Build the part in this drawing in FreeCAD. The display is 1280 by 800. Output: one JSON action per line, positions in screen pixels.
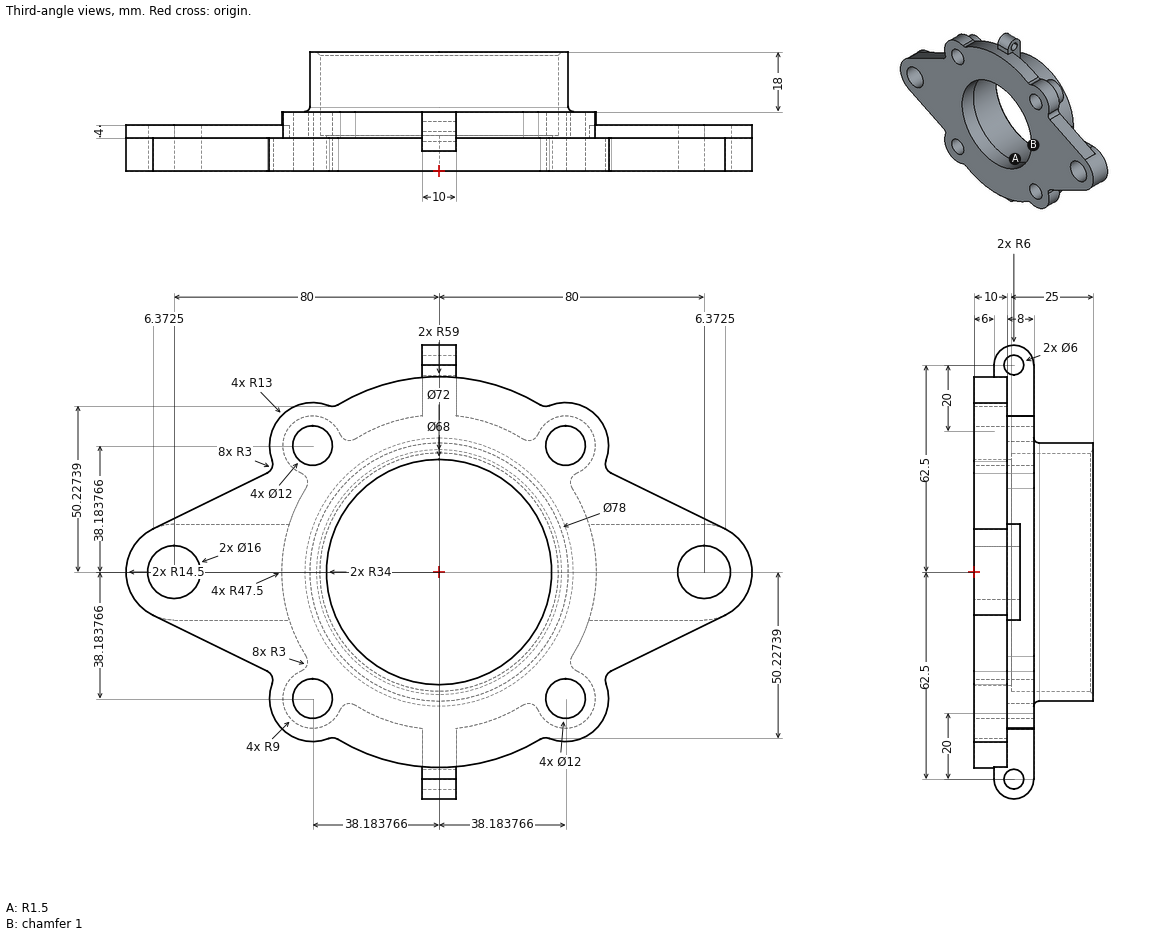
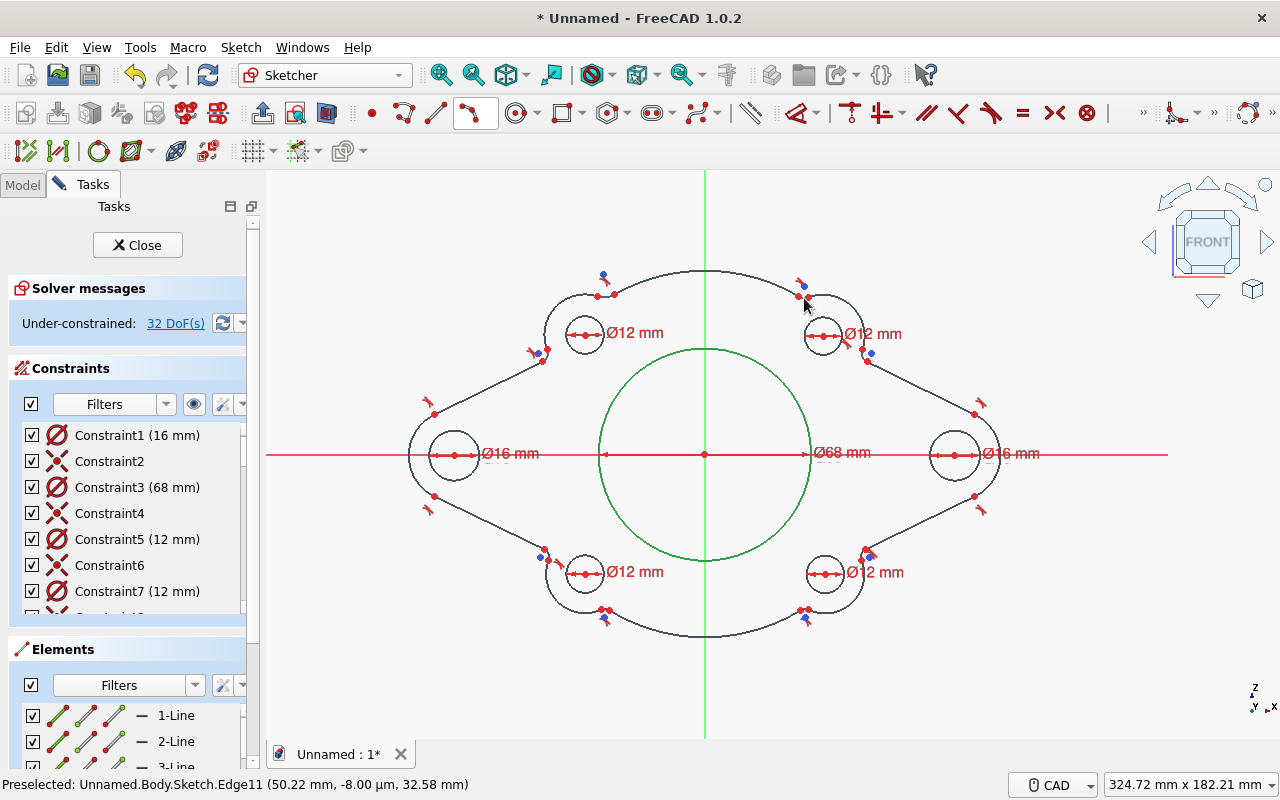
{"action": "scroll", "coordinate": [863, 552], "scroll_direction": "up", "scroll_amount": 7}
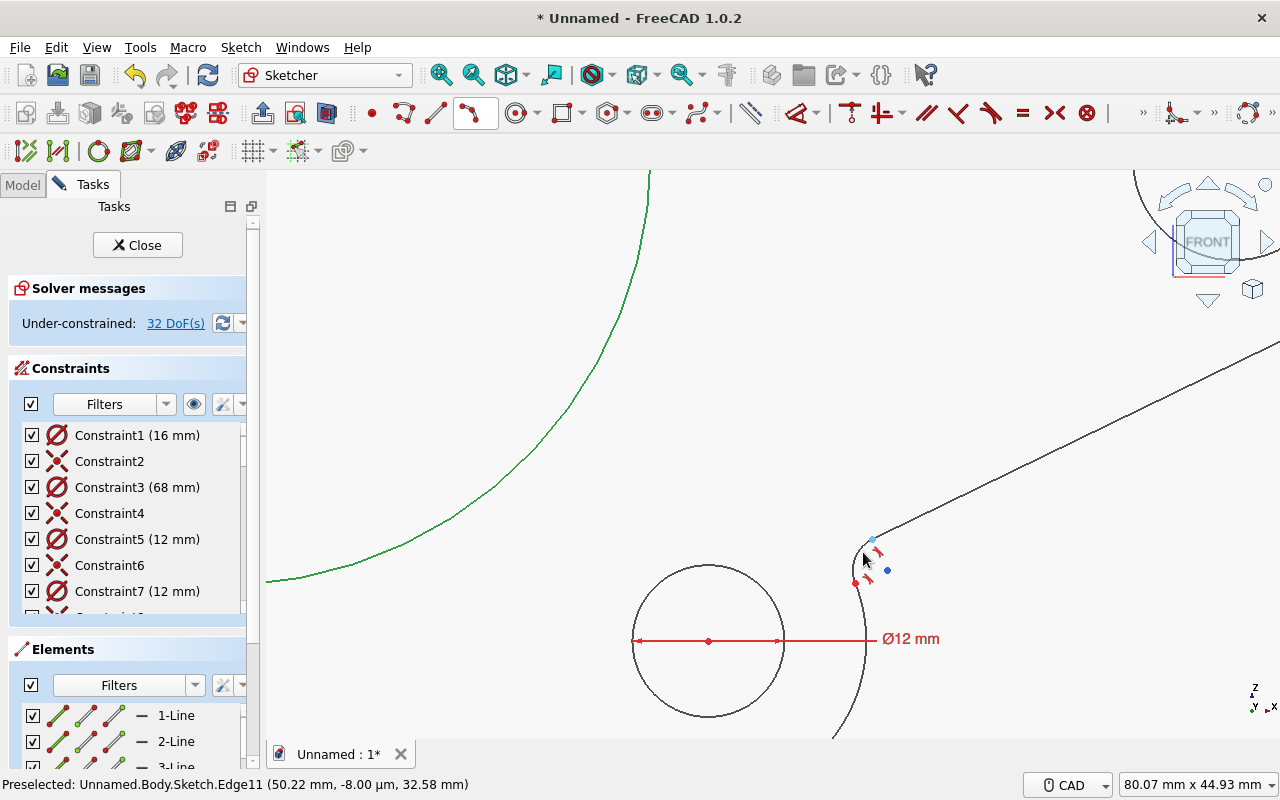
{"action": "left_click", "coordinate": [860, 549]}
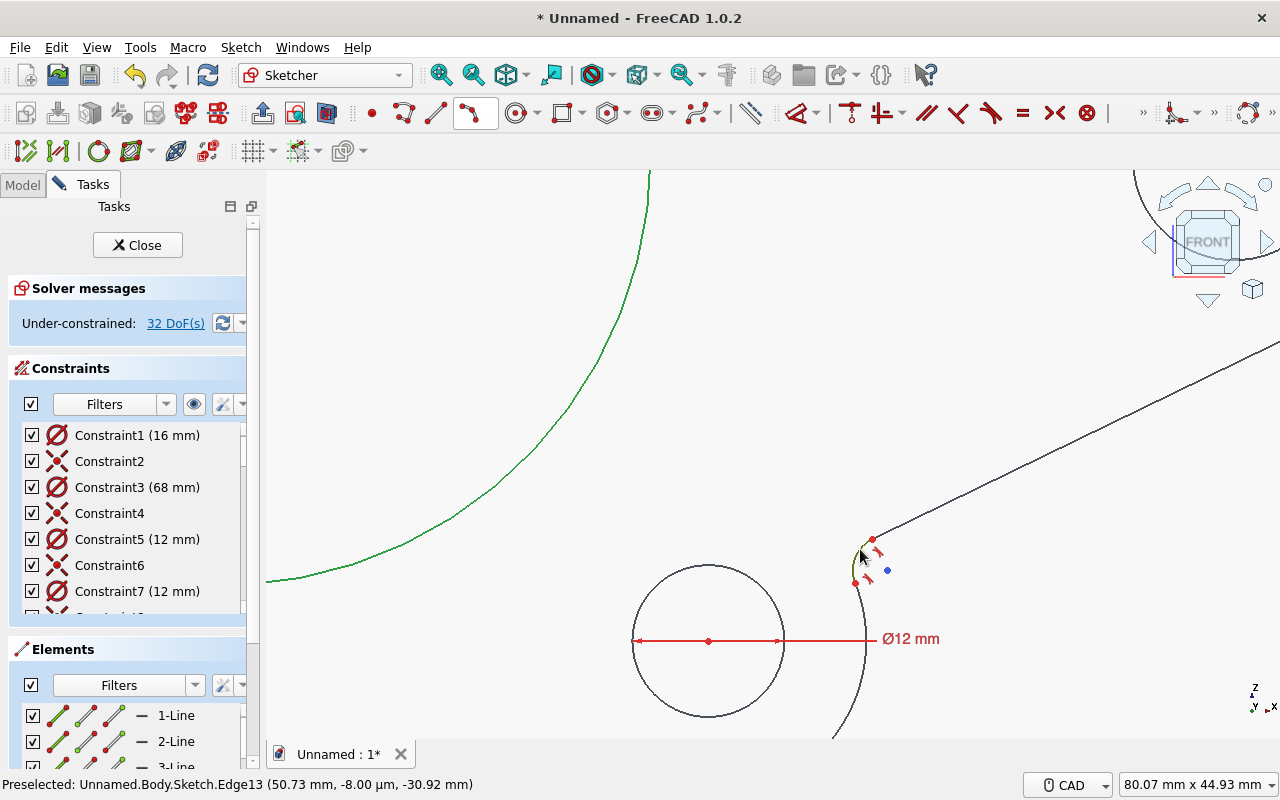
{"action": "scroll", "coordinate": [863, 553], "scroll_direction": "down", "scroll_amount": 7}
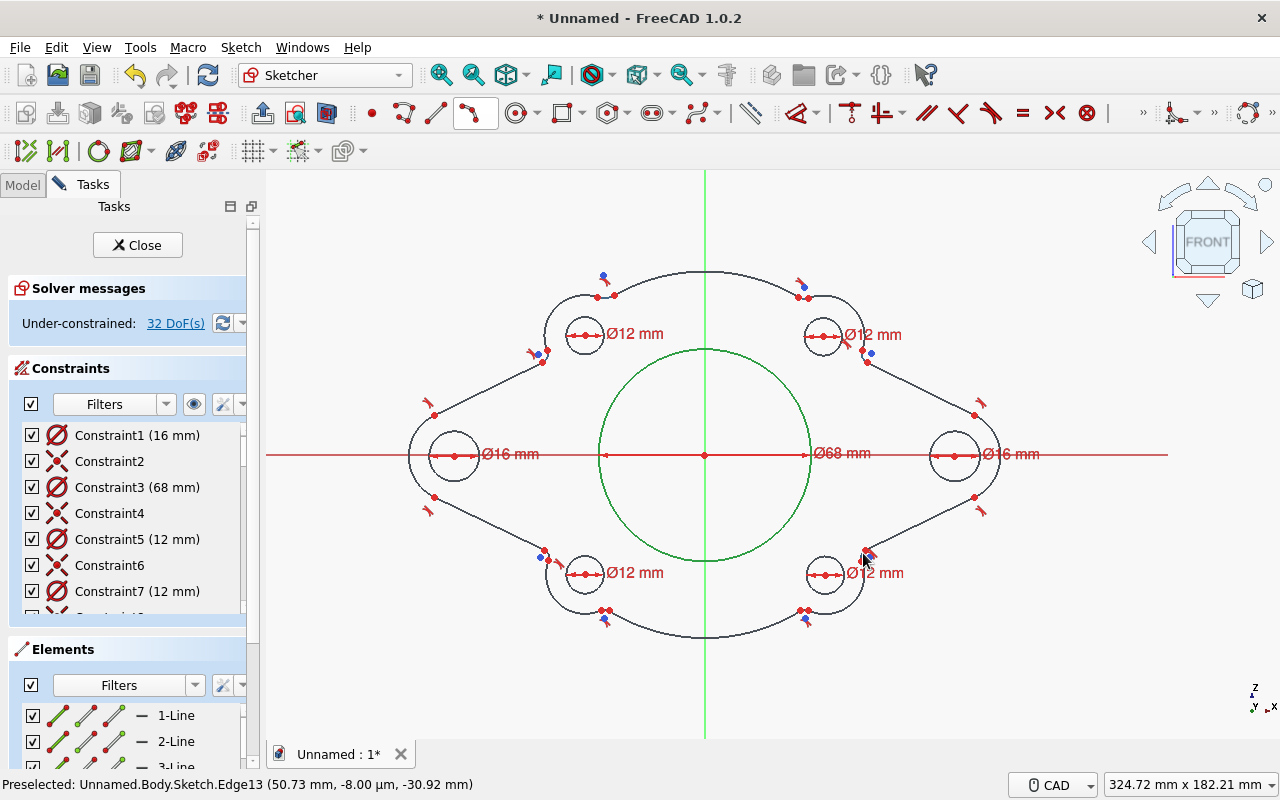
{"action": "scroll", "coordinate": [806, 610], "scroll_direction": "up", "scroll_amount": 9}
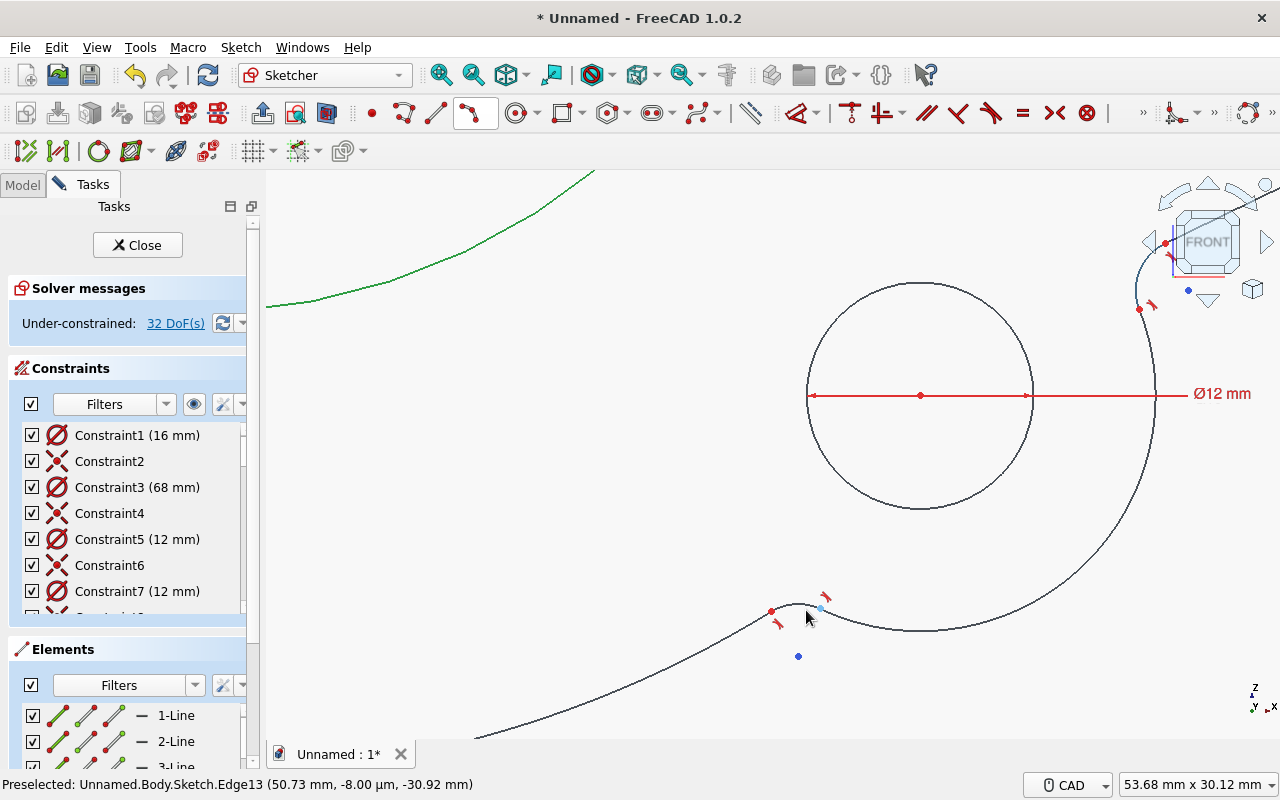
{"action": "left_click", "coordinate": [806, 605]}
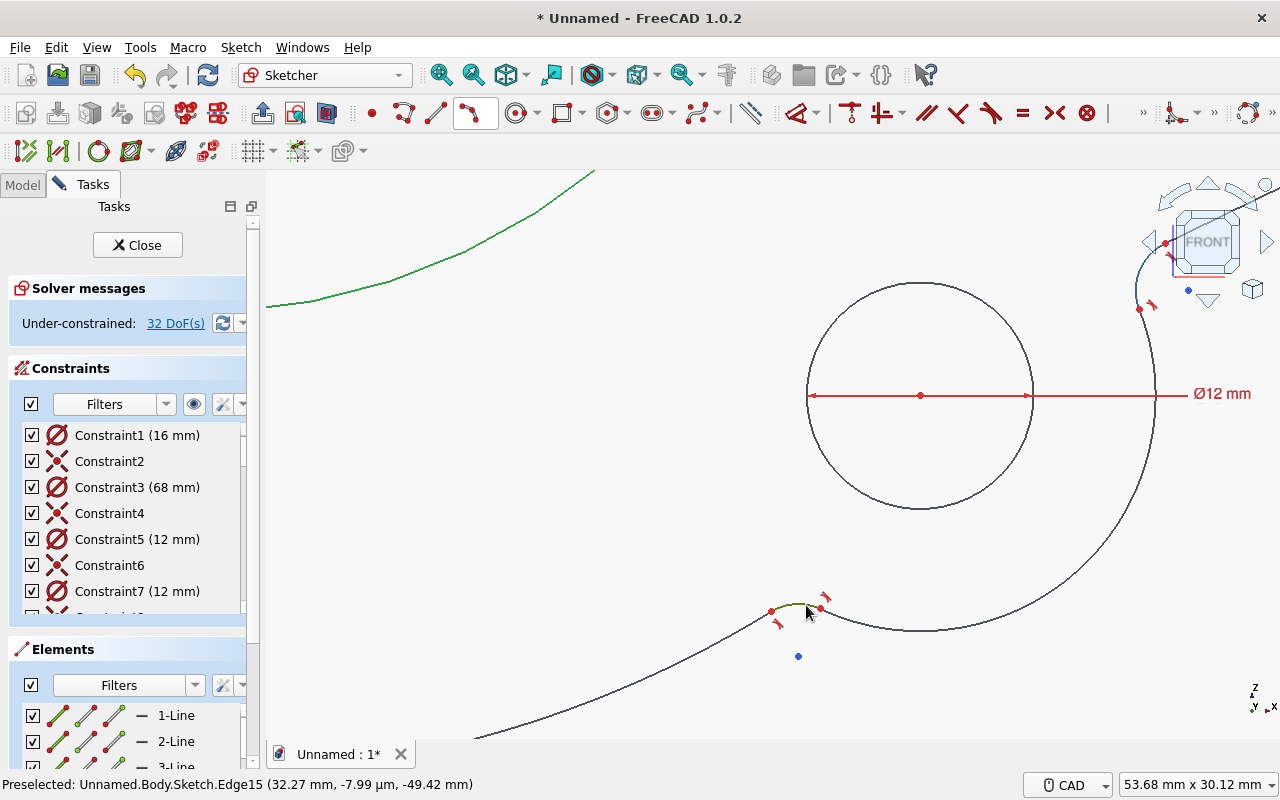
{"action": "scroll", "coordinate": [806, 610], "scroll_direction": "down", "scroll_amount": 9}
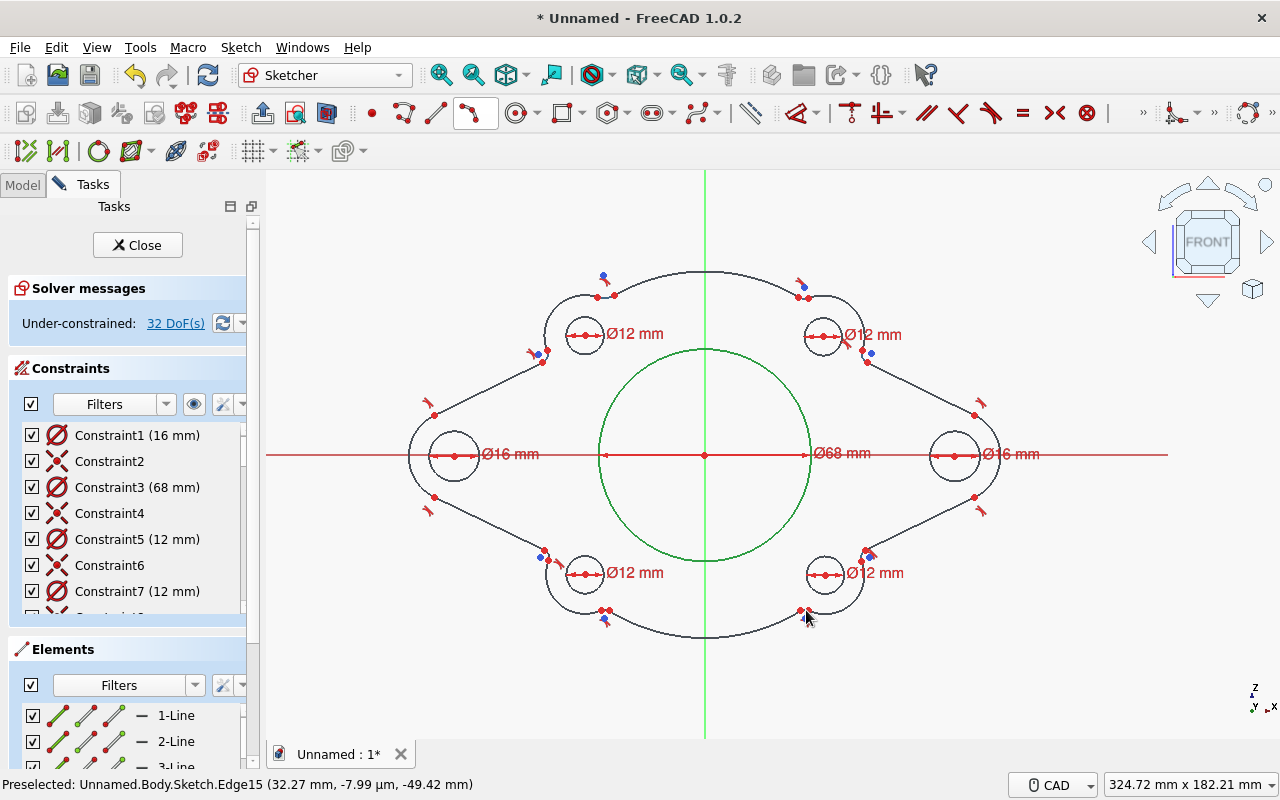
{"action": "scroll", "coordinate": [607, 610], "scroll_direction": "up", "scroll_amount": 9}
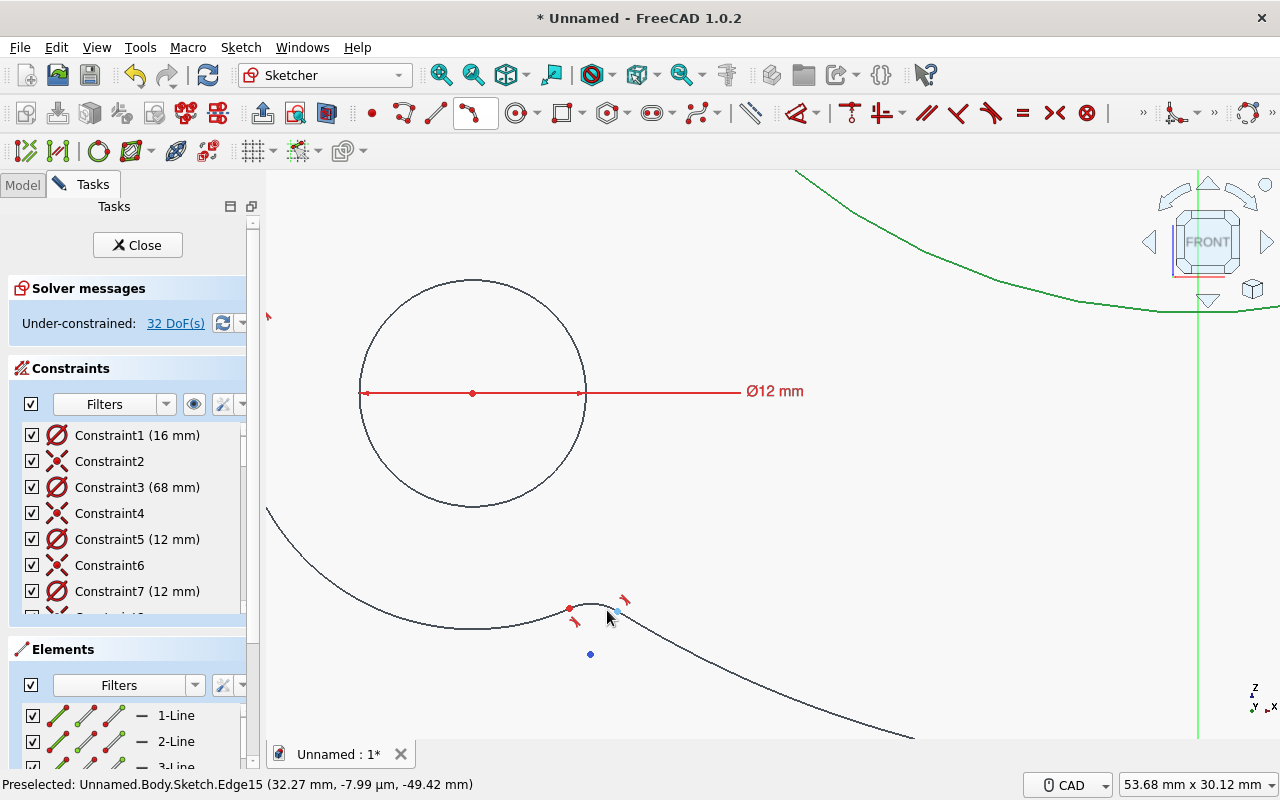
{"action": "left_click", "coordinate": [604, 606]}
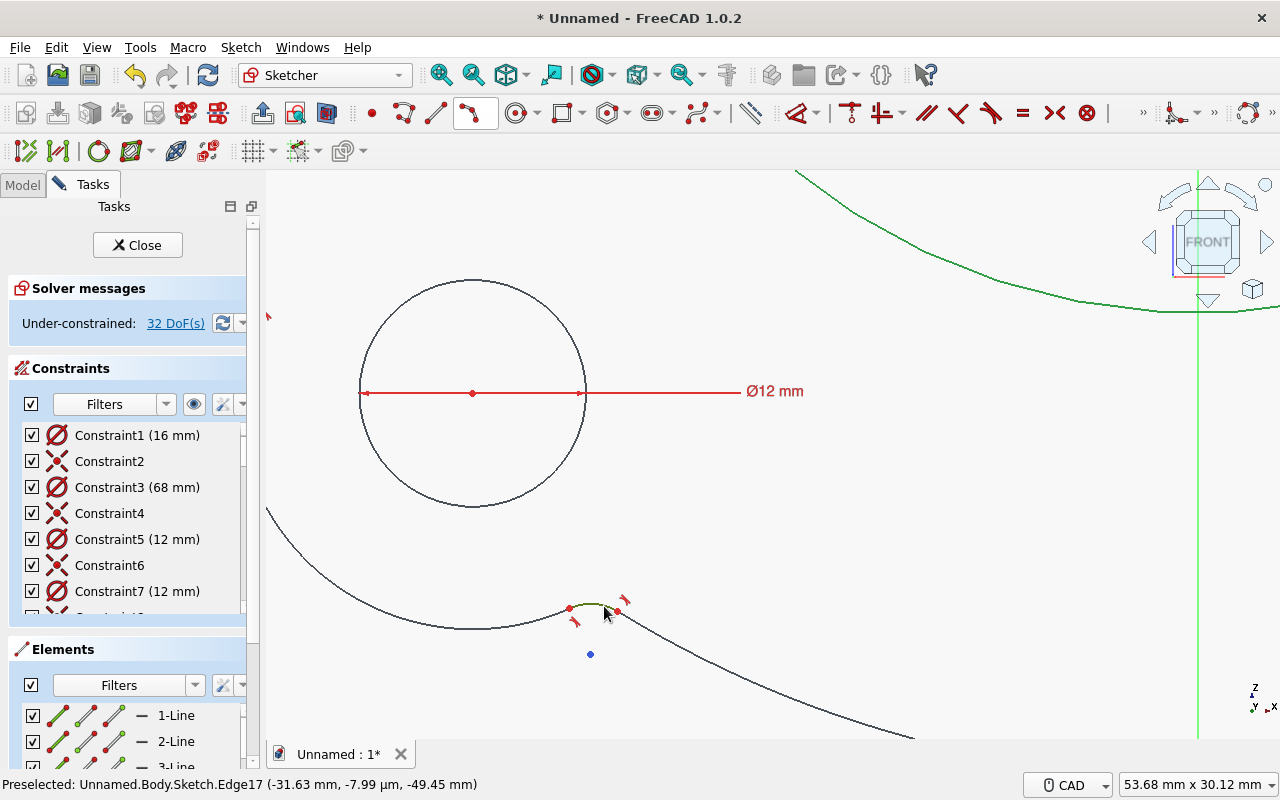
{"action": "scroll", "coordinate": [607, 610], "scroll_direction": "down", "scroll_amount": 9}